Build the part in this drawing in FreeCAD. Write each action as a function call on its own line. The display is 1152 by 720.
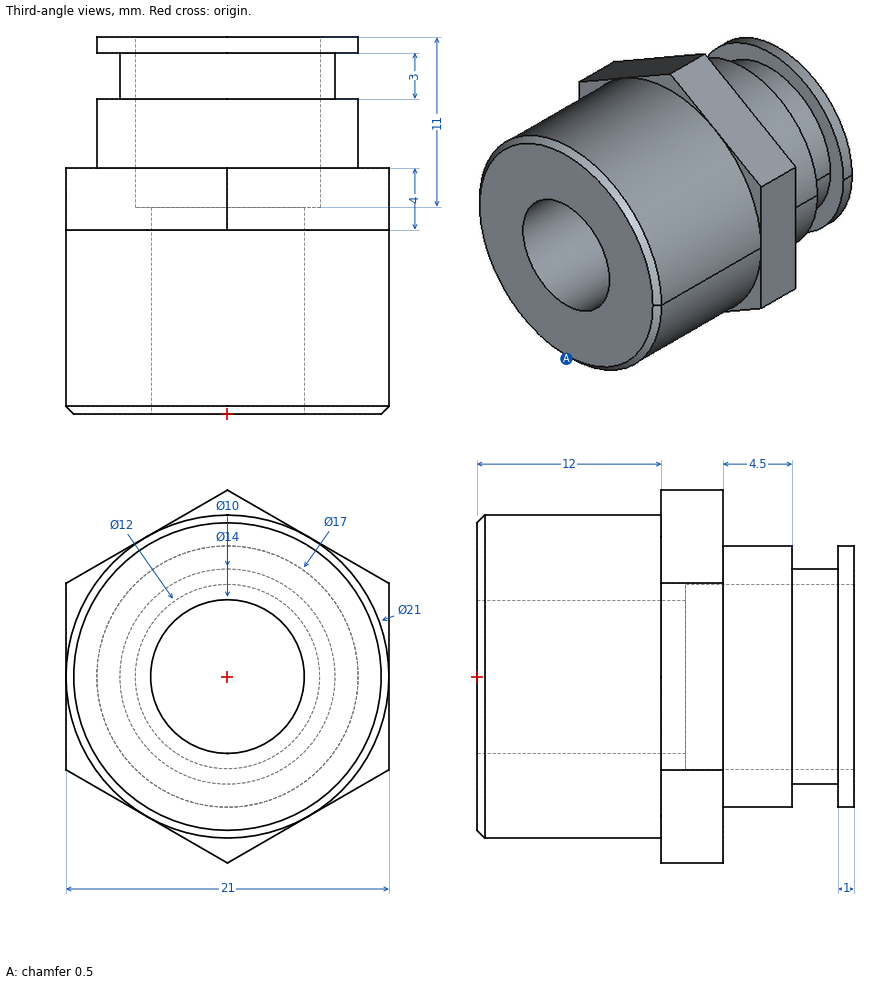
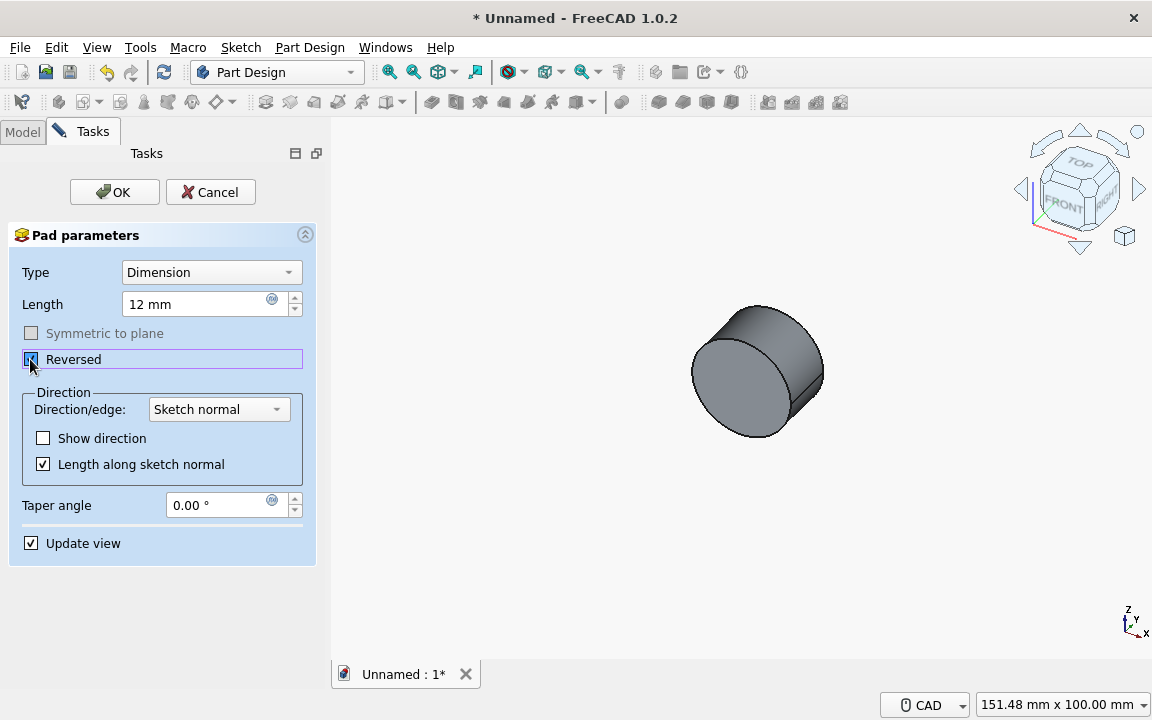
click(115, 192)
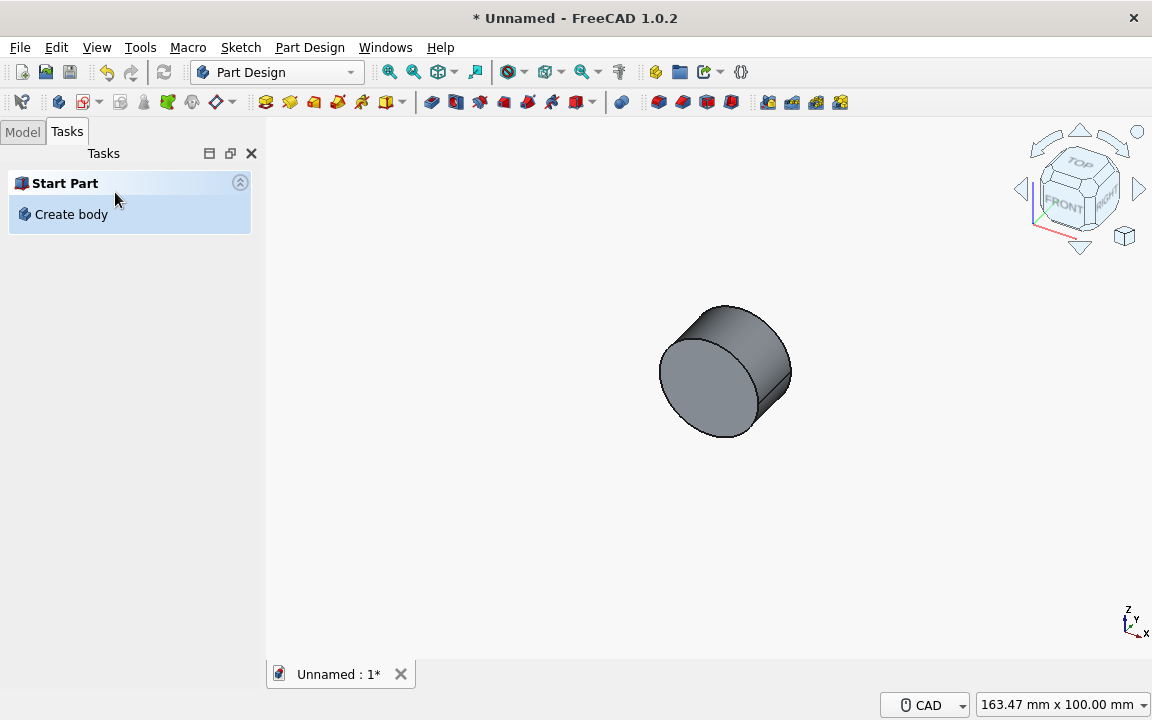
key(v)
key(f)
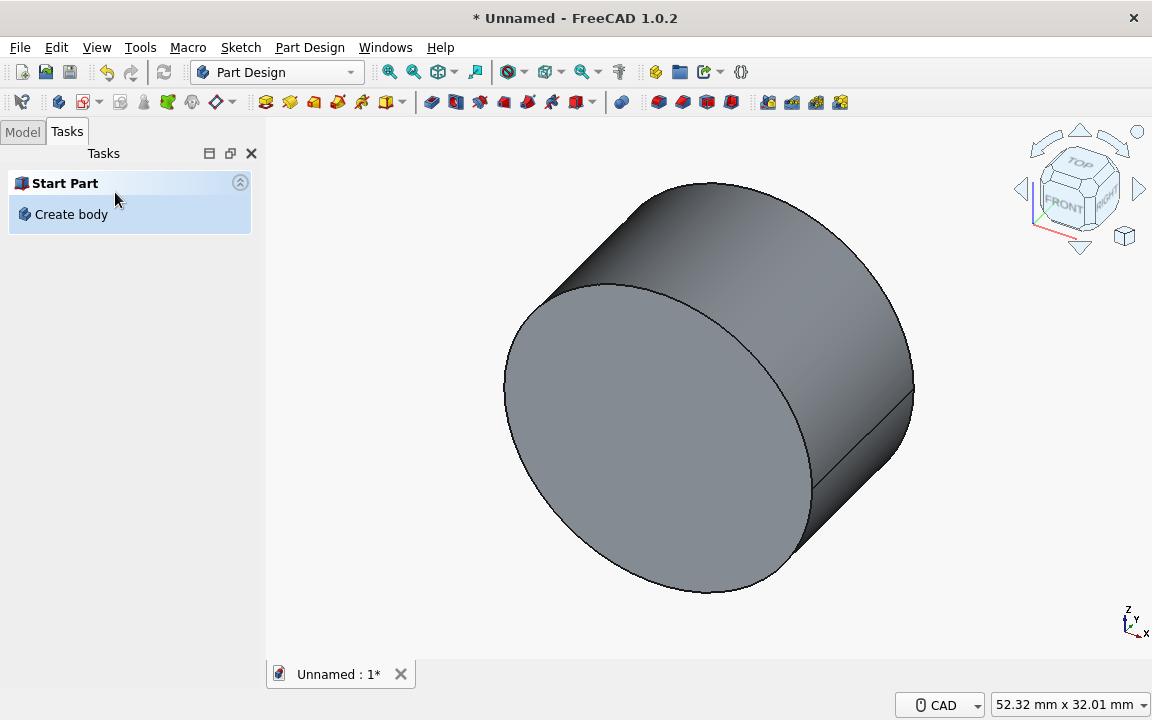
key(4)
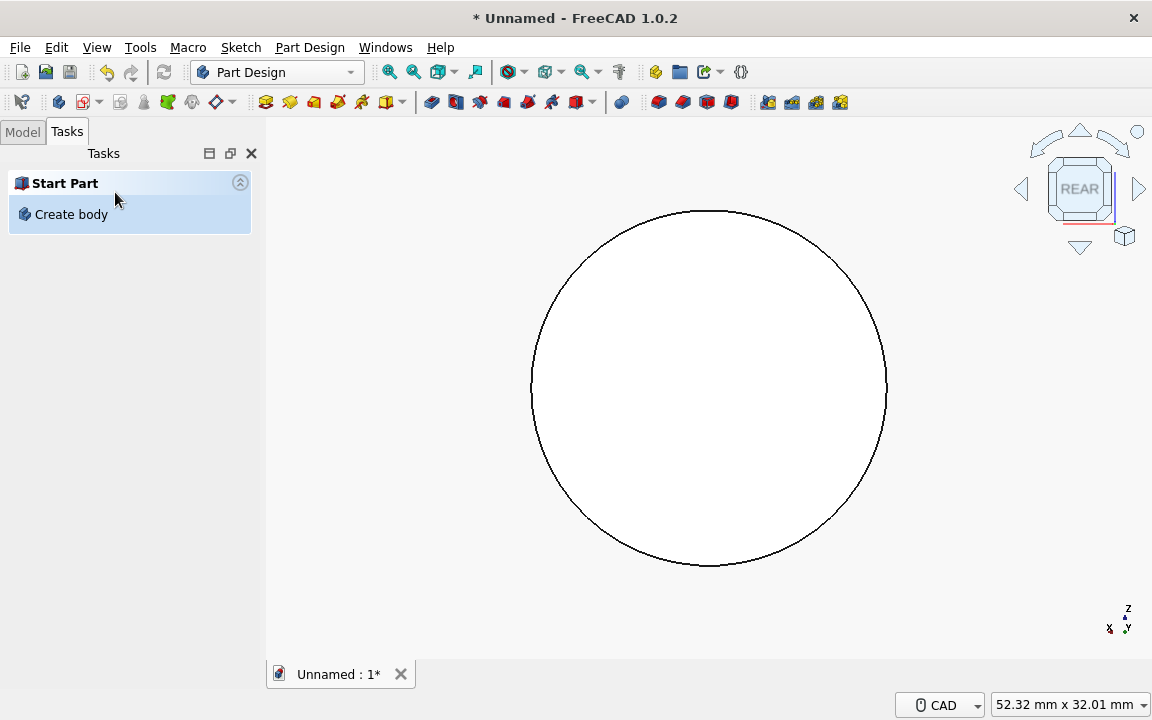
click(709, 387)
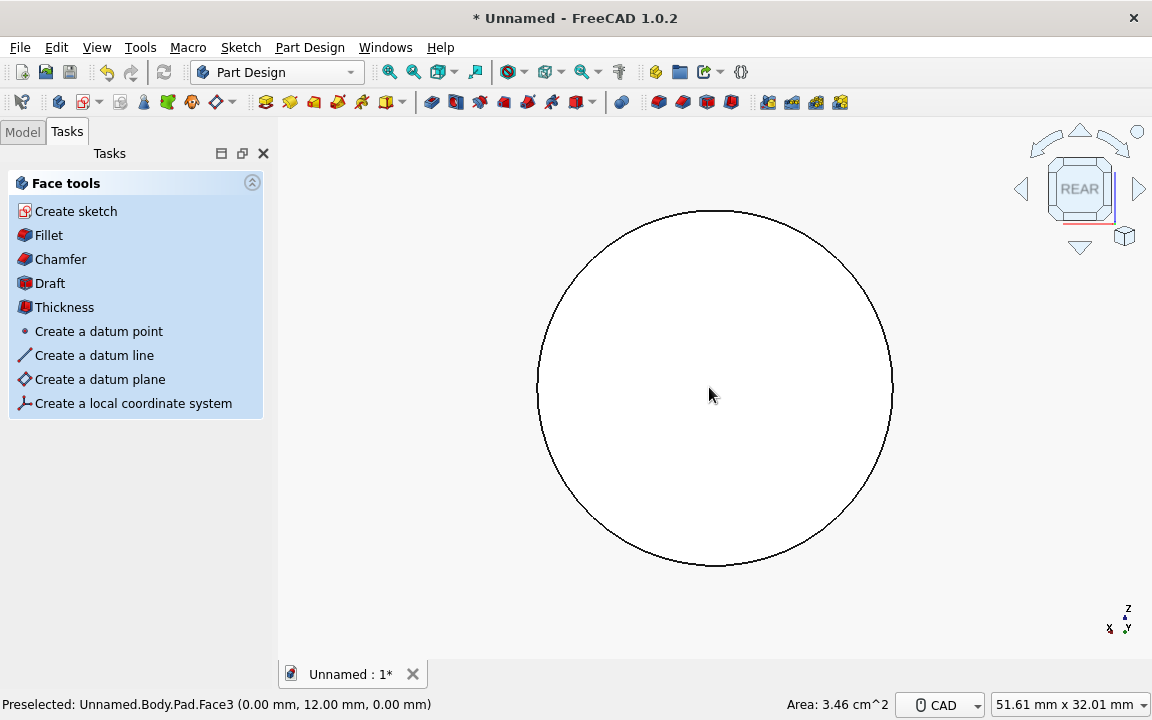
click(84, 102)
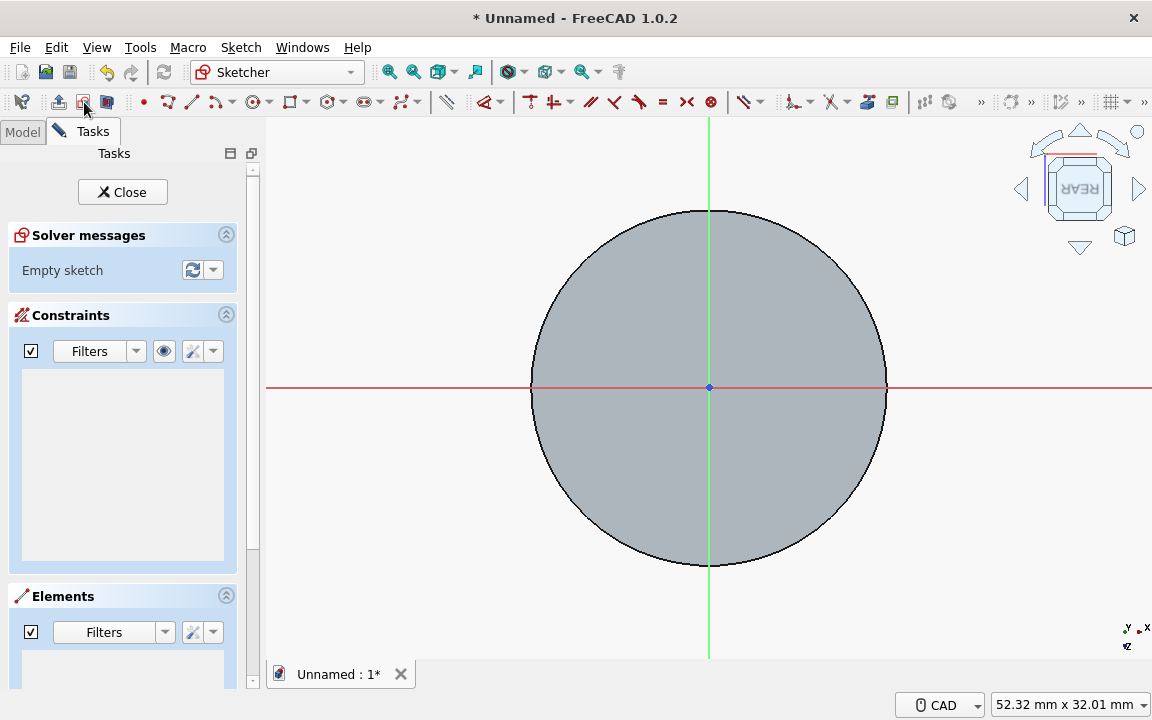
key(g)
key(p)
key(6)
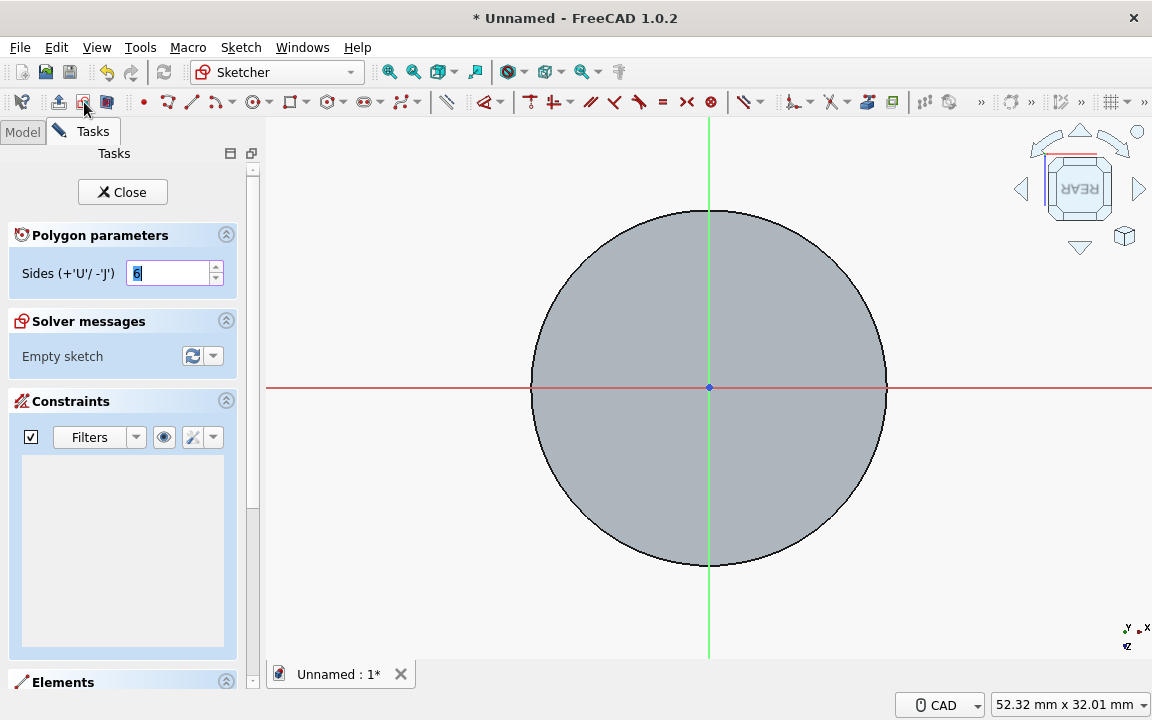
click(709, 388)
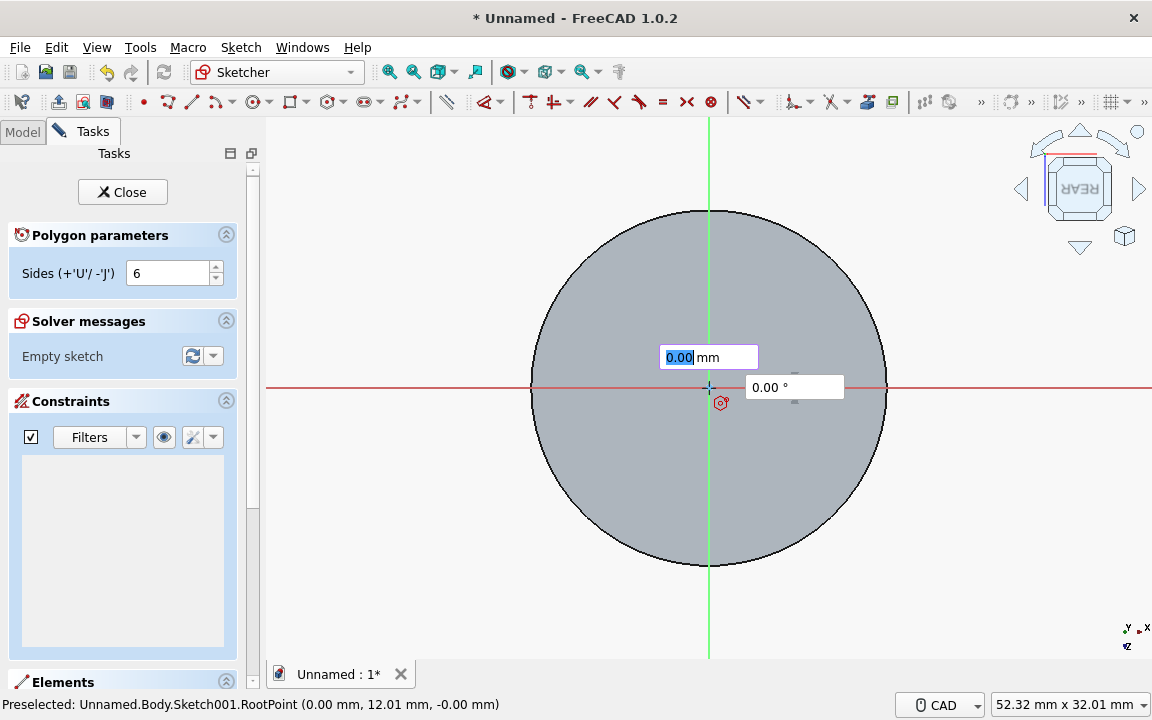
click(709, 183)
right_click(709, 183)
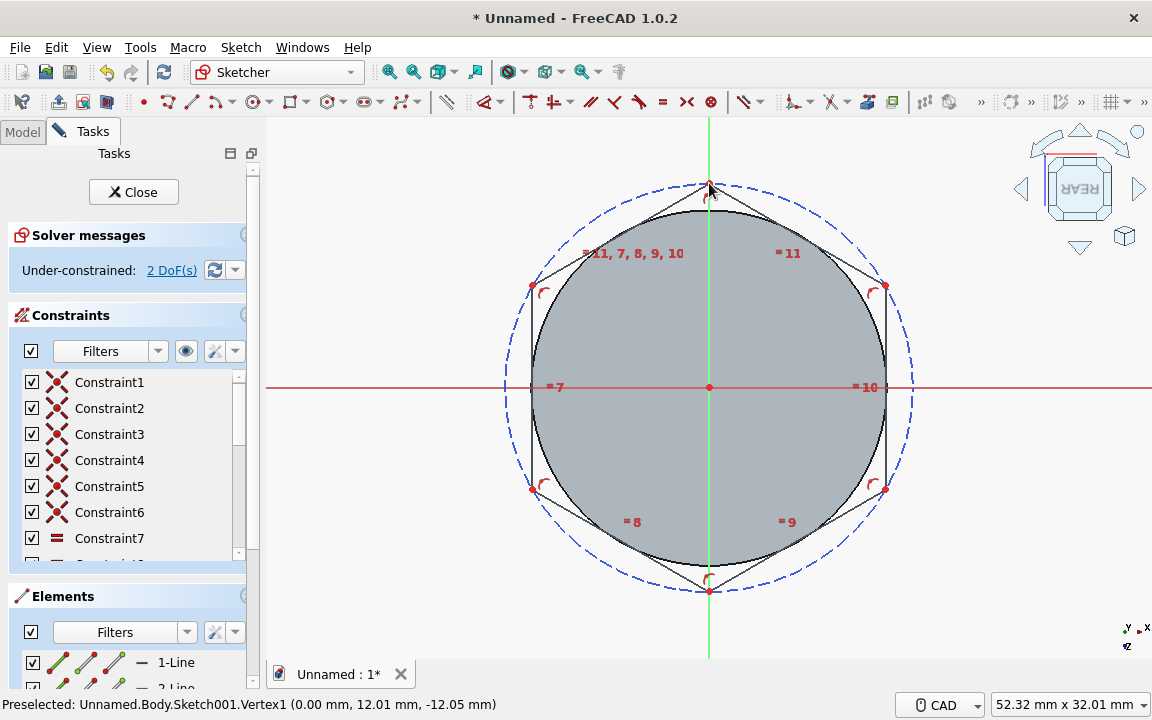
click(532, 347)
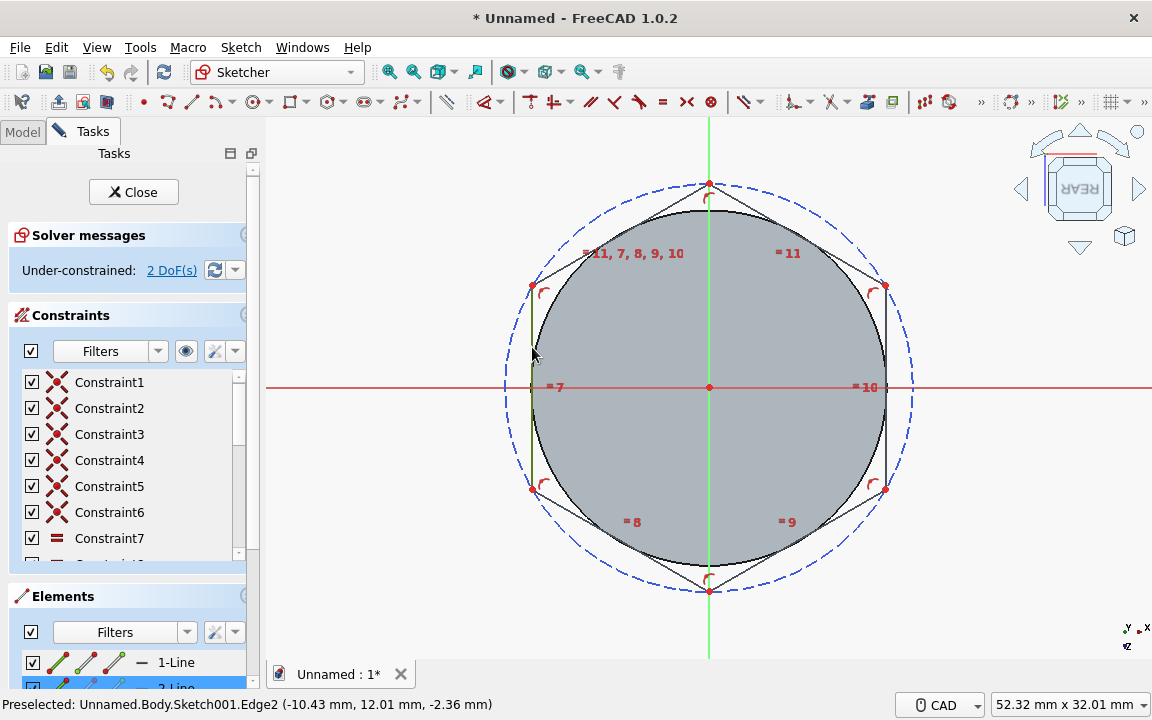
key(v)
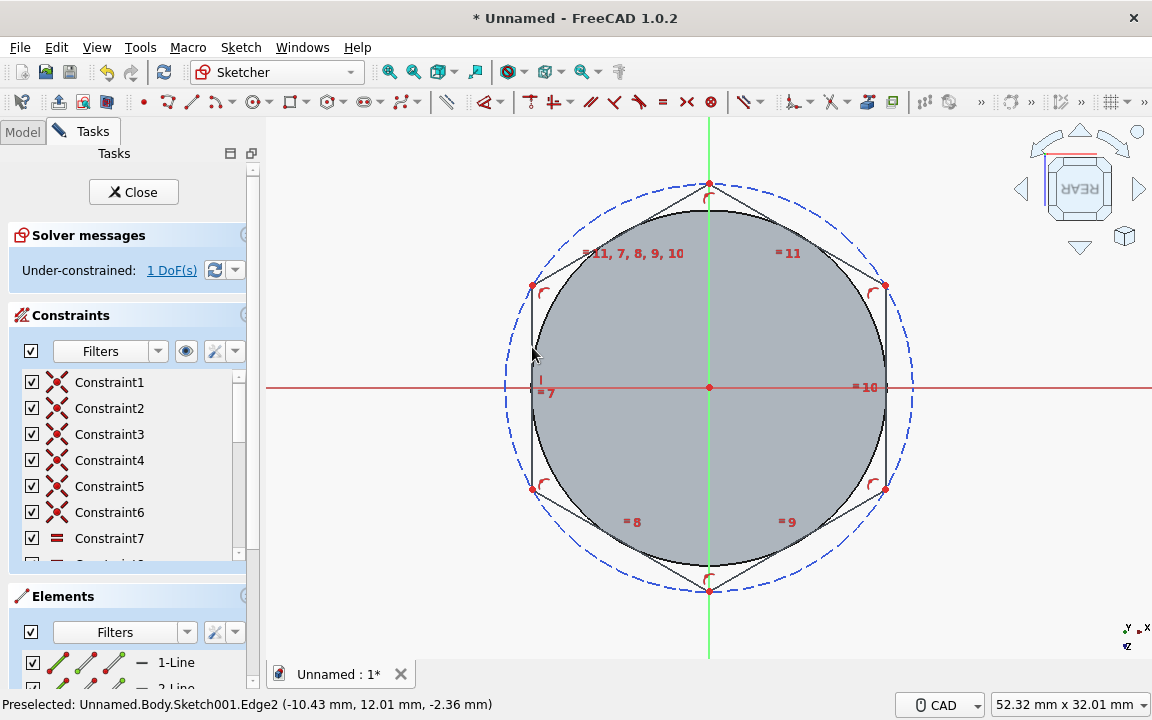
key(d)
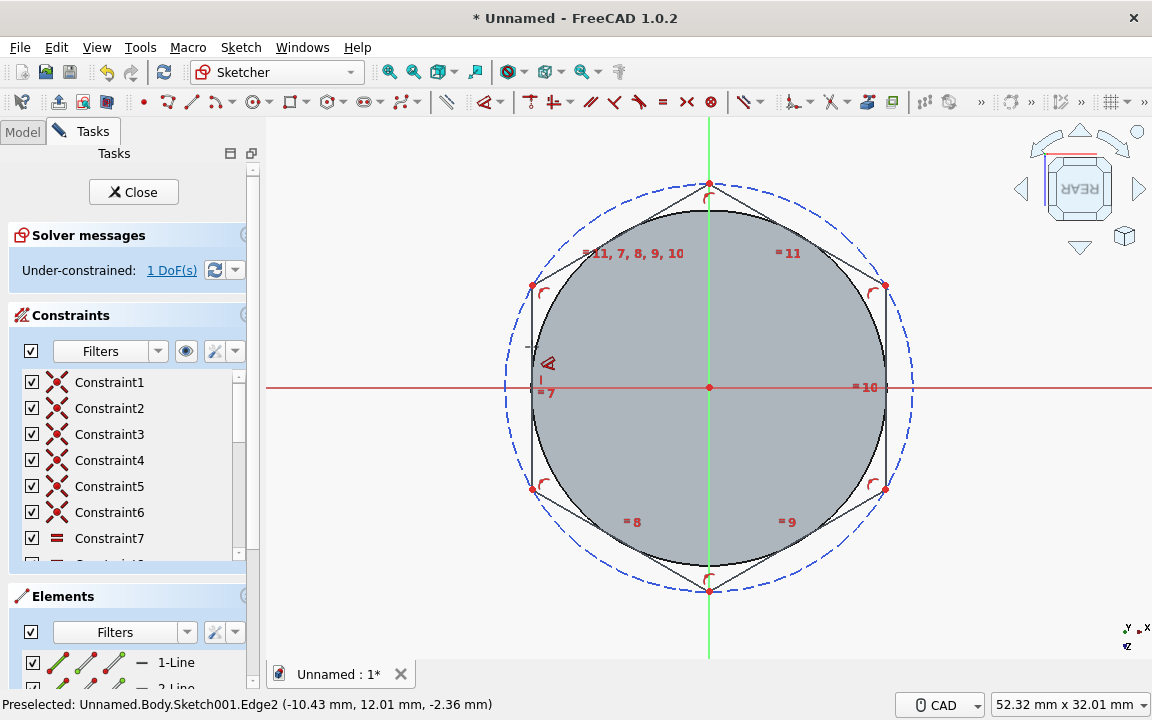
click(532, 286)